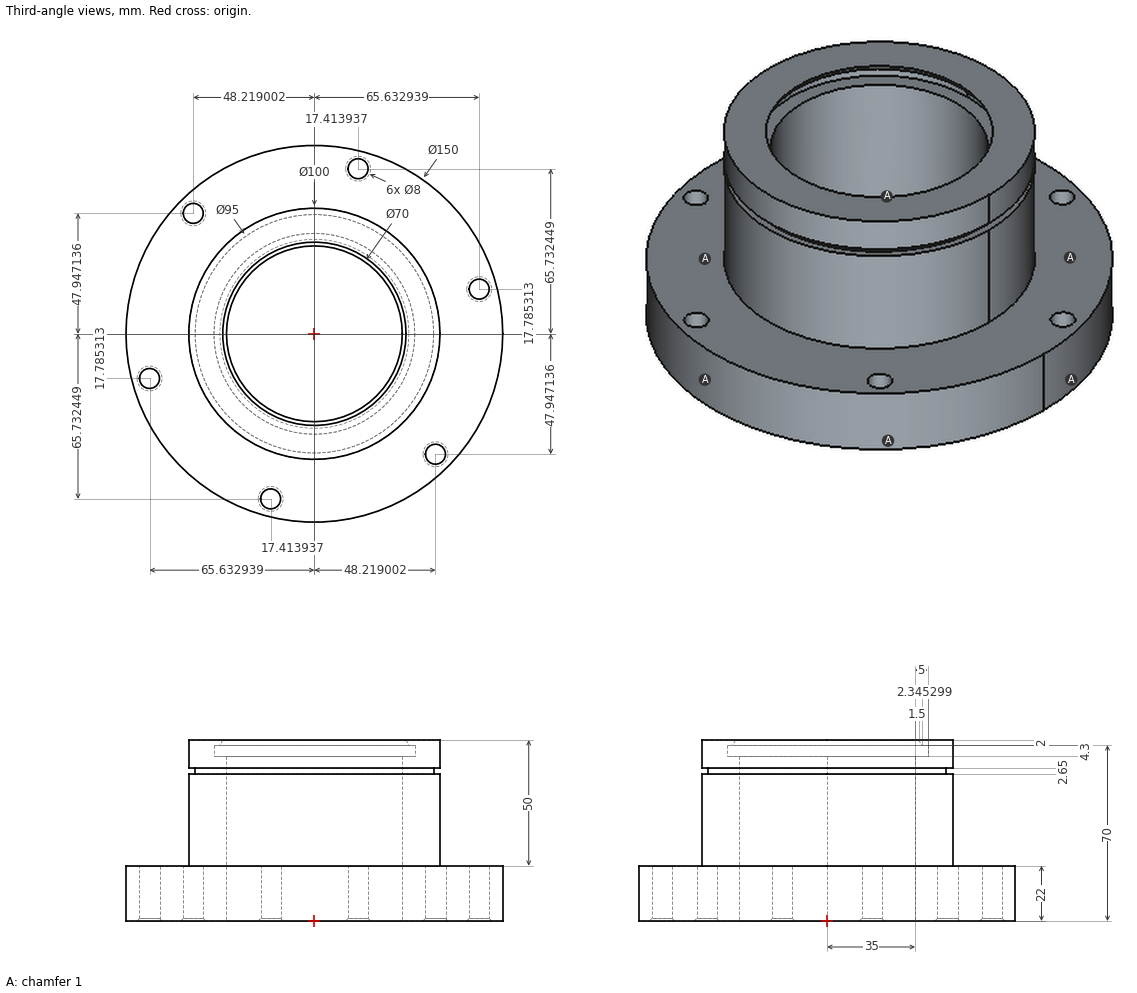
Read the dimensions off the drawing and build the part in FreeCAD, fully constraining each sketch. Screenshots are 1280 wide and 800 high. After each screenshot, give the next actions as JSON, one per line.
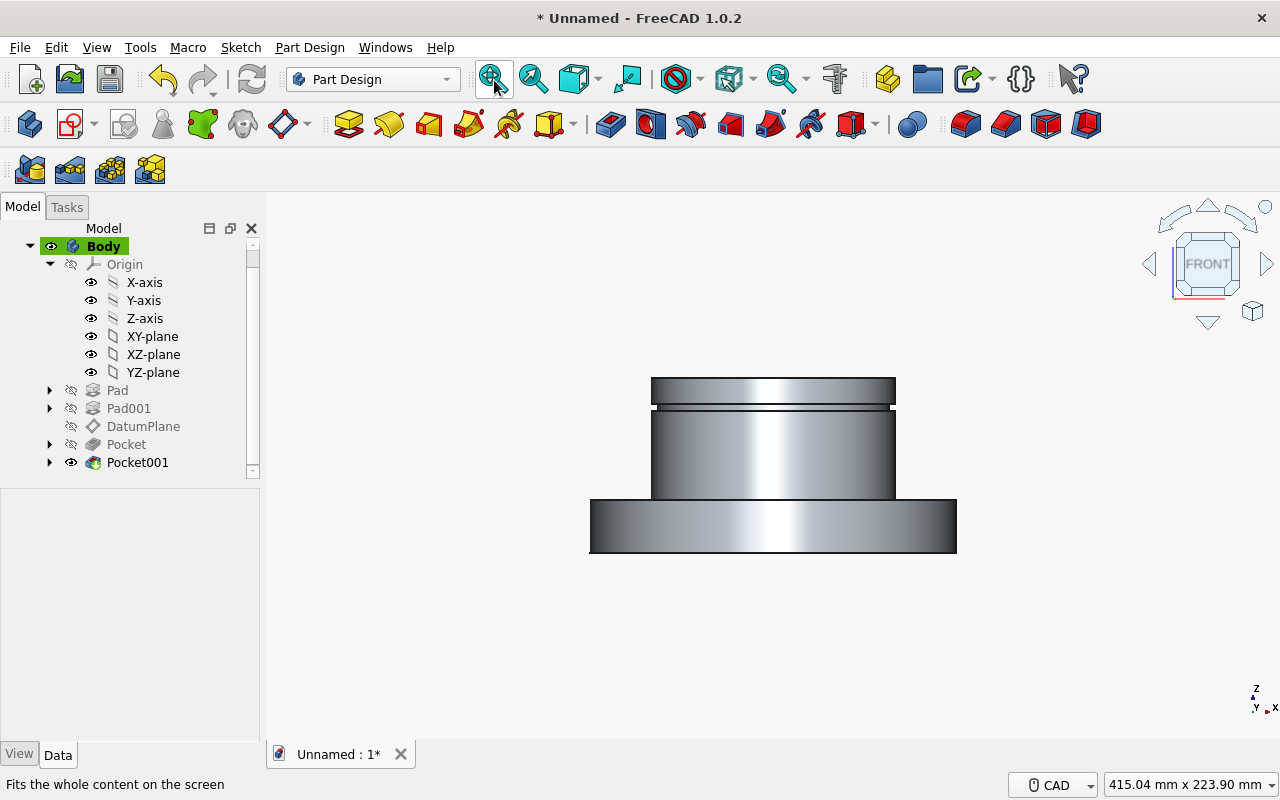
{"action": "key", "text": "3"}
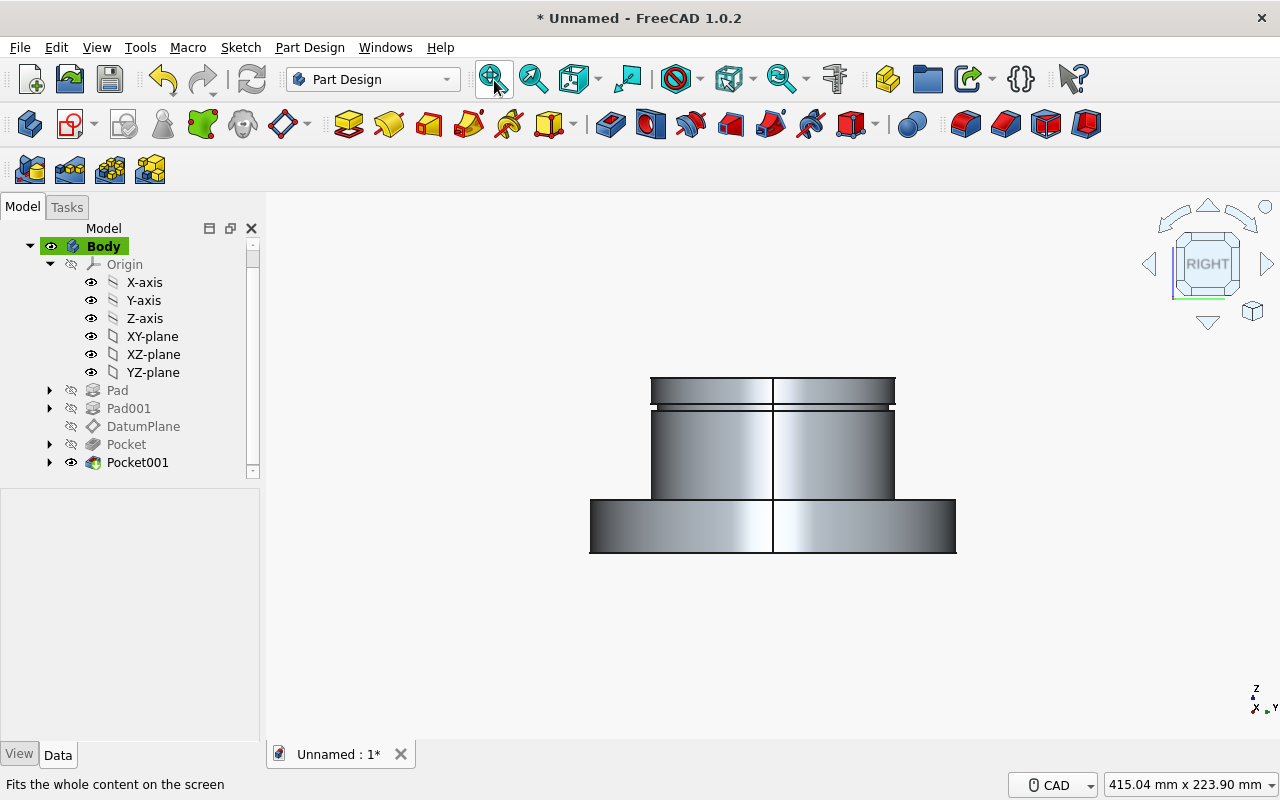
{"action": "left_click", "coordinate": [494, 80]}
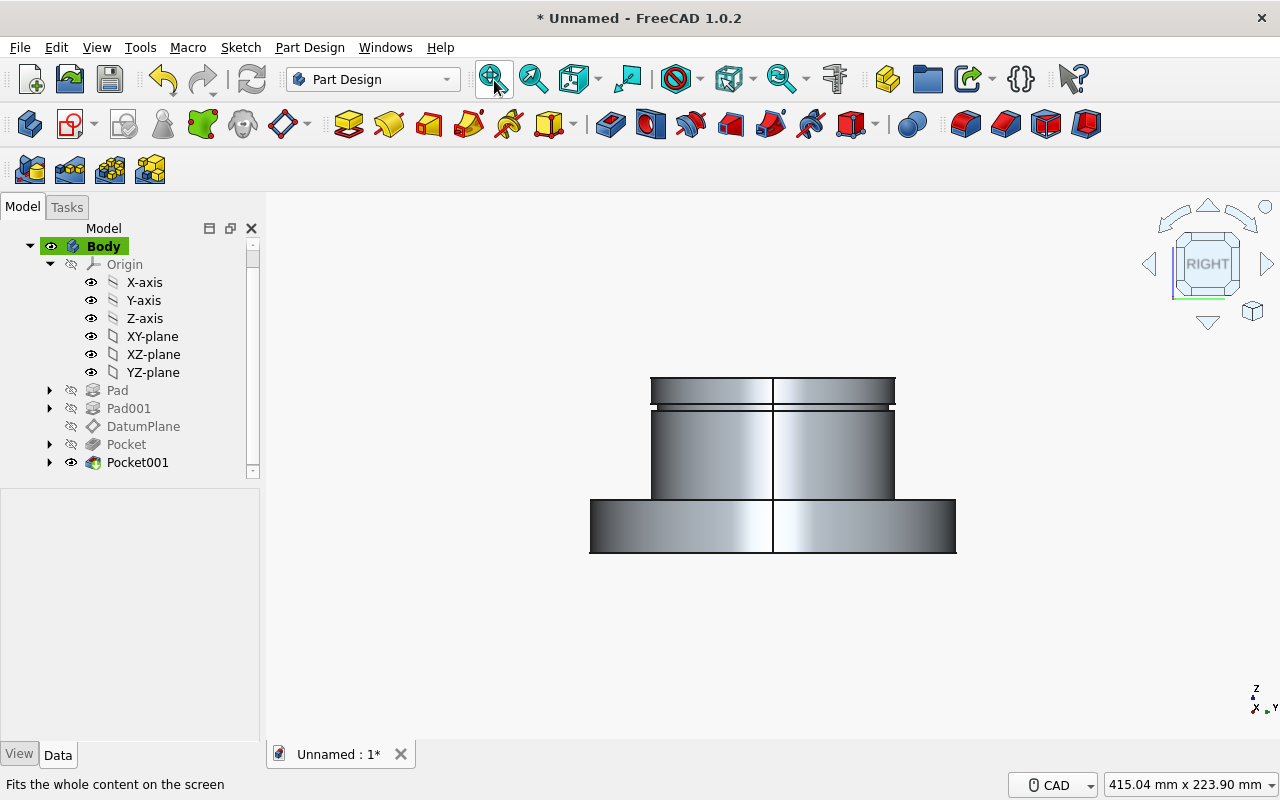
{"action": "key", "text": "5"}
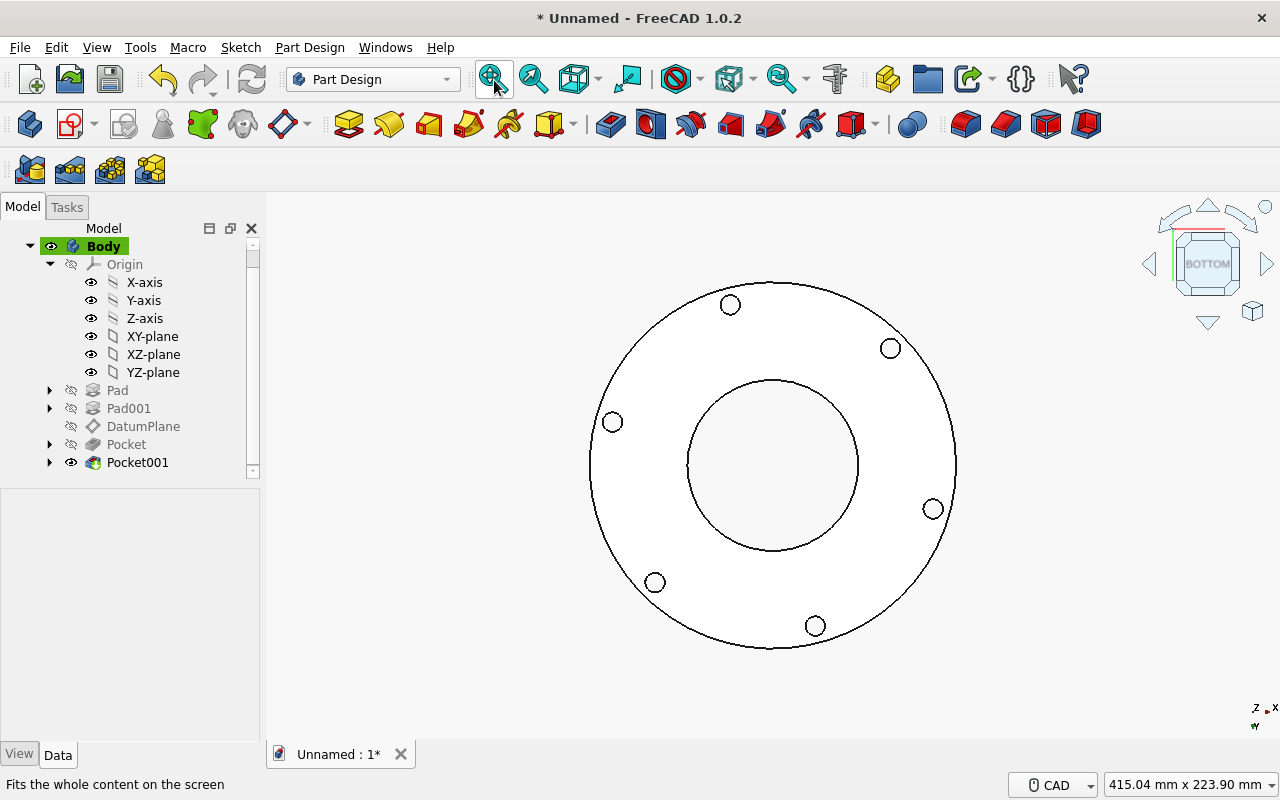
{"action": "left_click", "coordinate": [806, 625]}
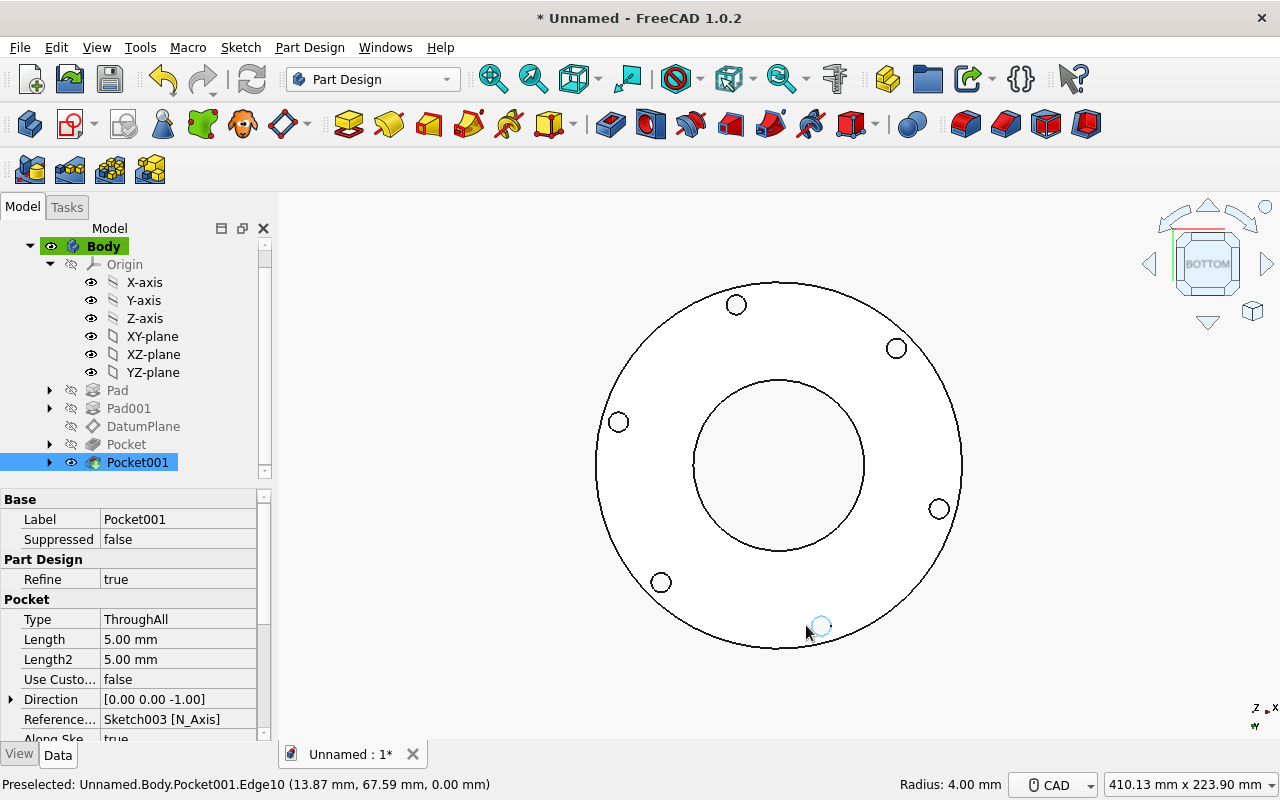
{"action": "left_click", "coordinate": [651, 582], "text": "ctrl"}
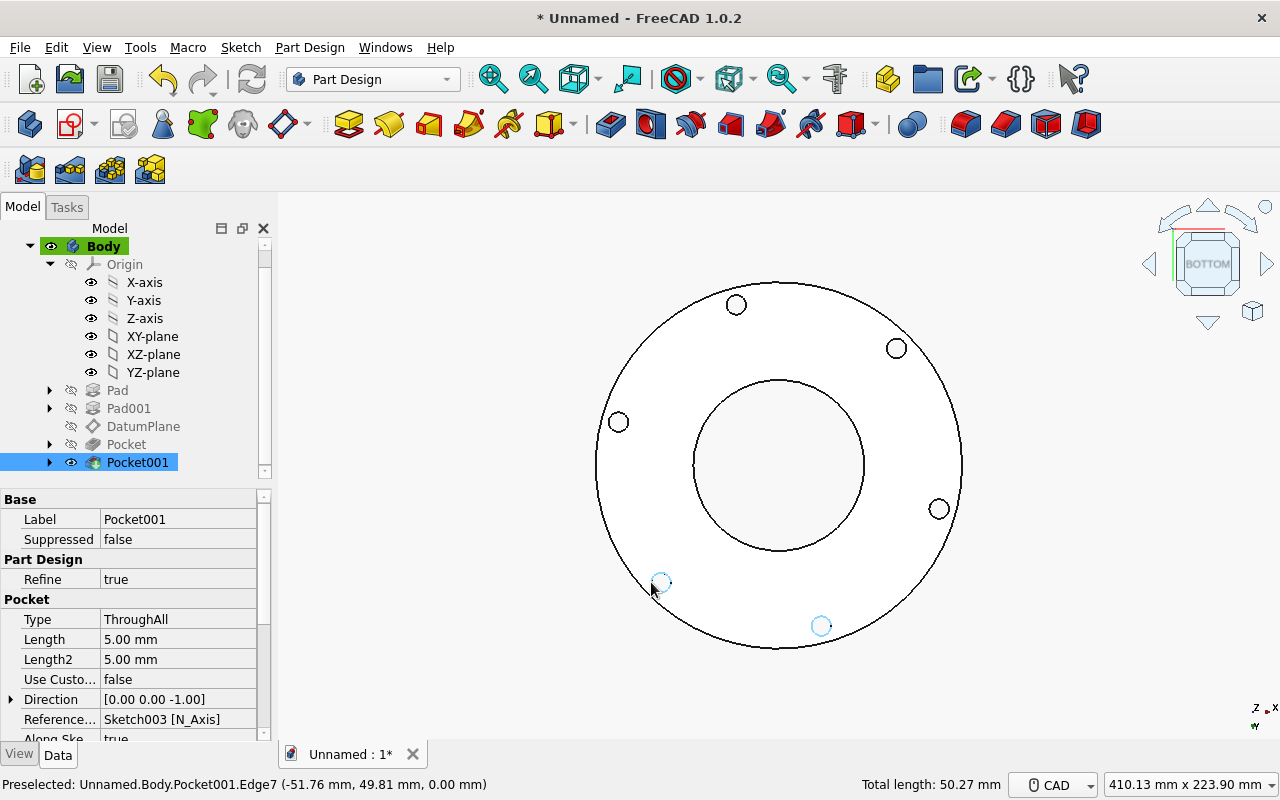
{"action": "left_click", "coordinate": [611, 427], "text": "ctrl"}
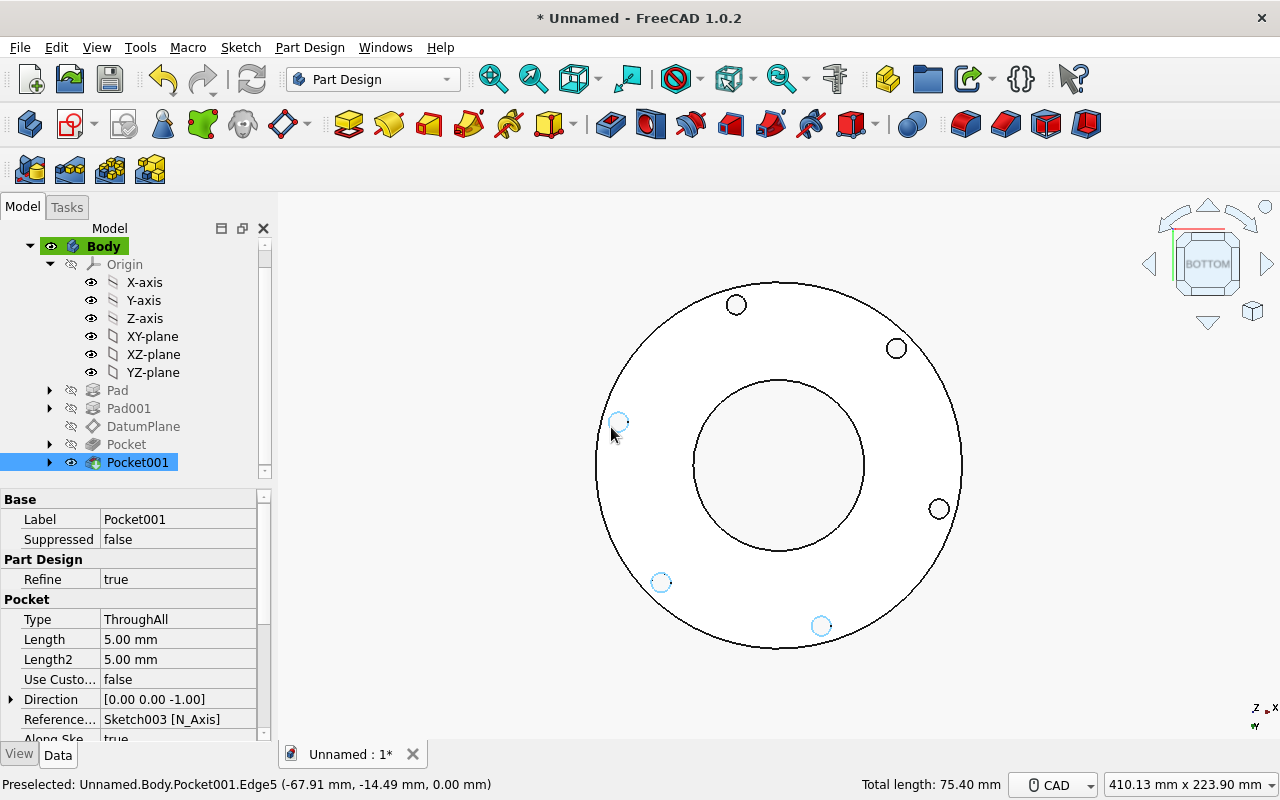
{"action": "left_click", "coordinate": [727, 304], "text": "ctrl"}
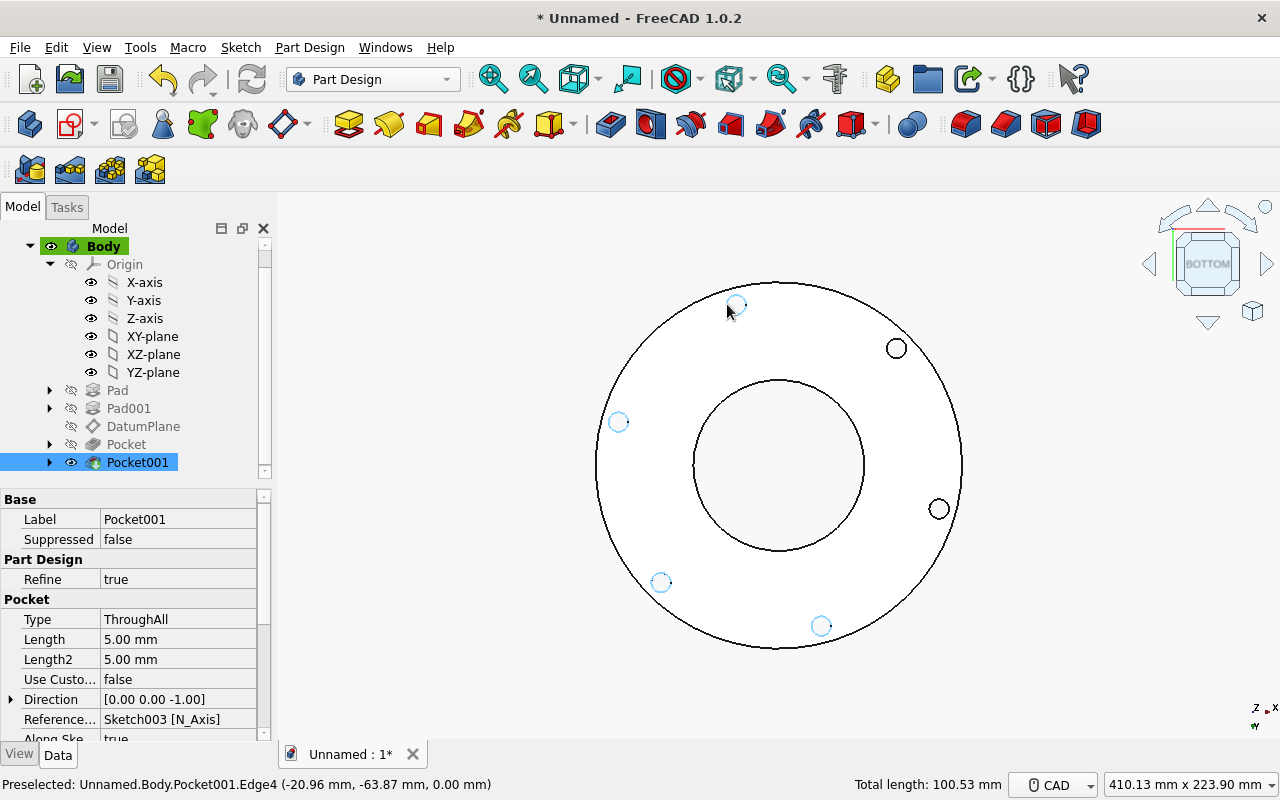
{"action": "left_click", "coordinate": [887, 347], "text": "ctrl"}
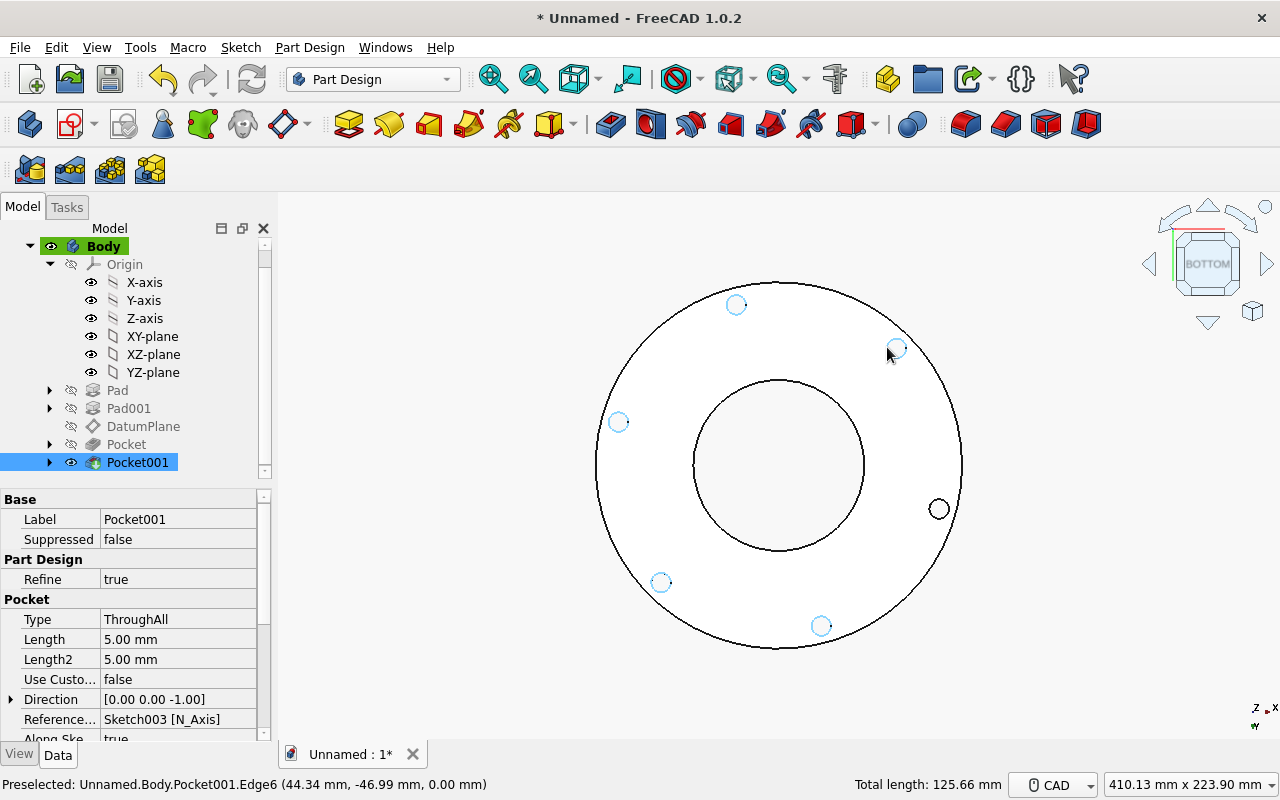
{"action": "left_click", "coordinate": [931, 514], "text": "ctrl"}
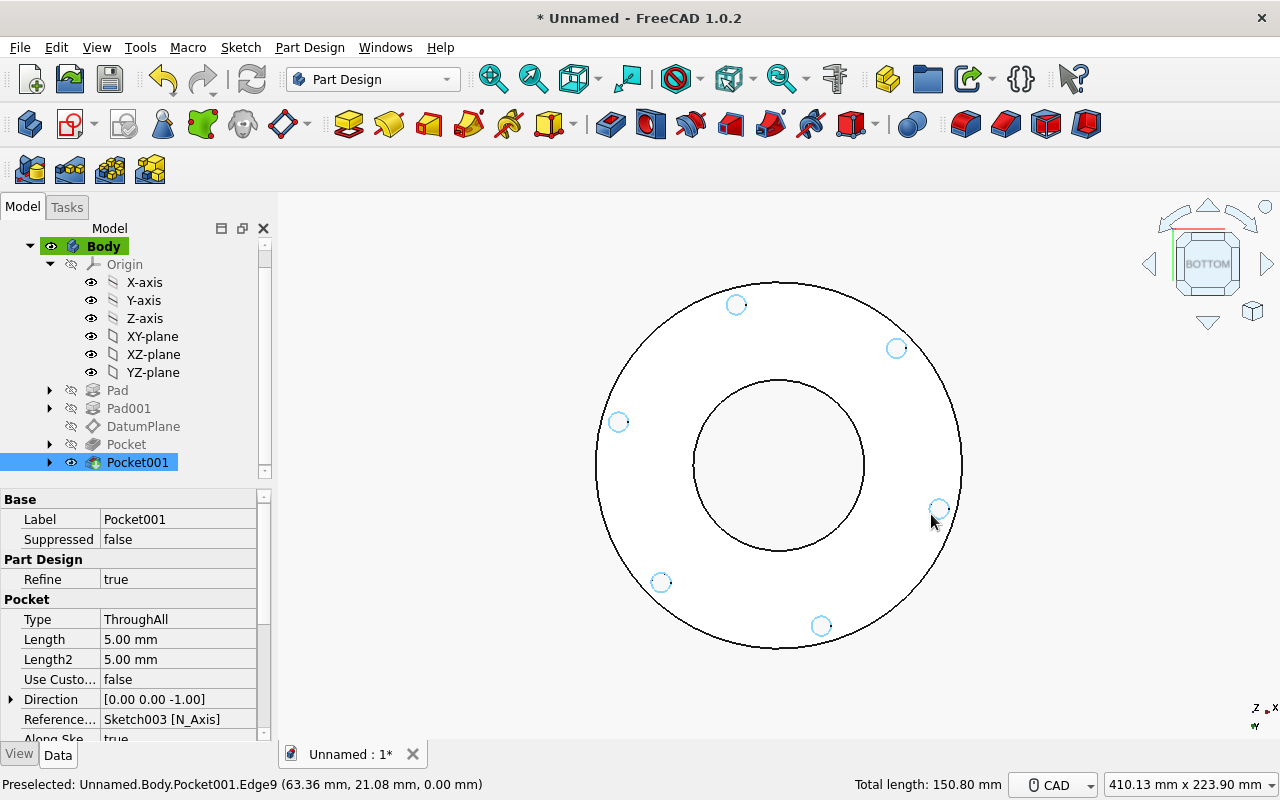
{"action": "left_click", "coordinate": [1006, 124]}